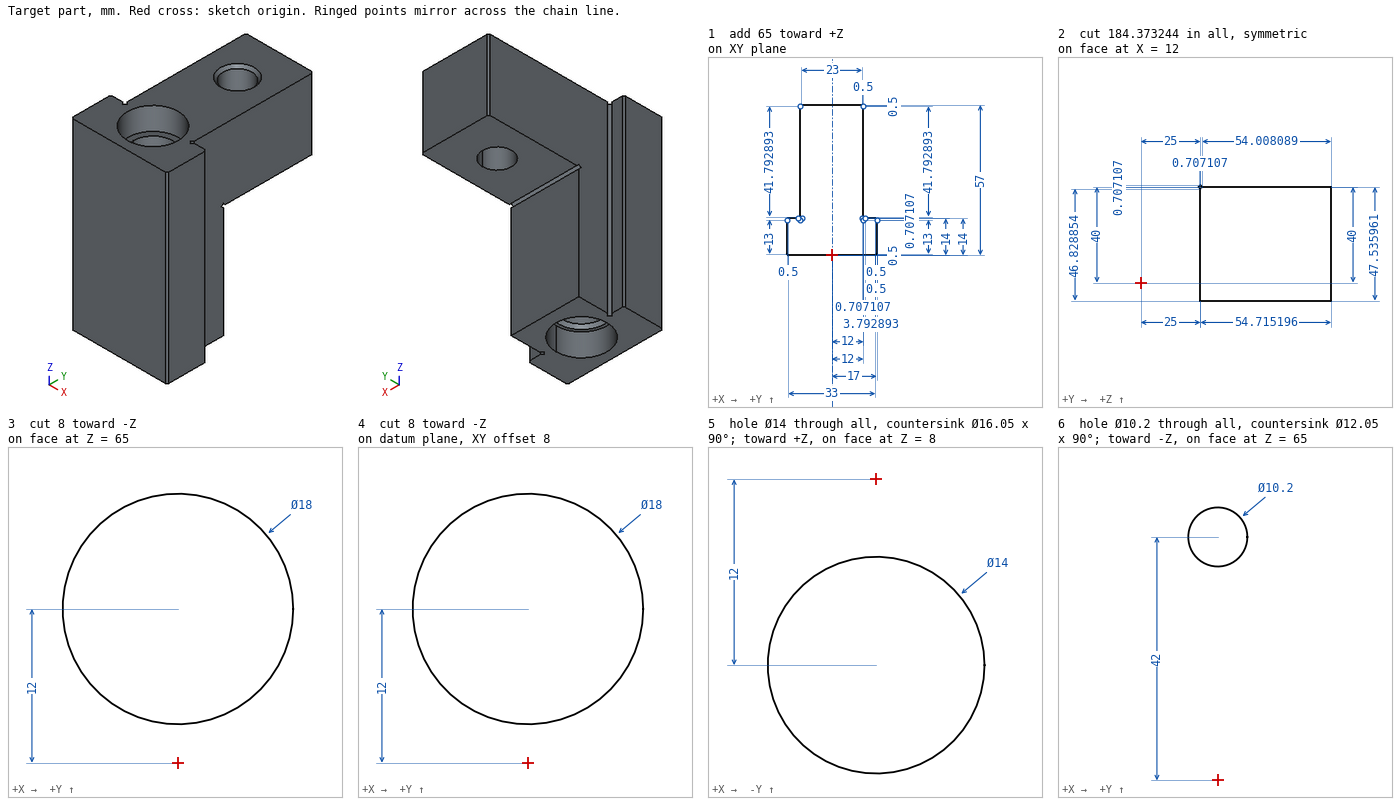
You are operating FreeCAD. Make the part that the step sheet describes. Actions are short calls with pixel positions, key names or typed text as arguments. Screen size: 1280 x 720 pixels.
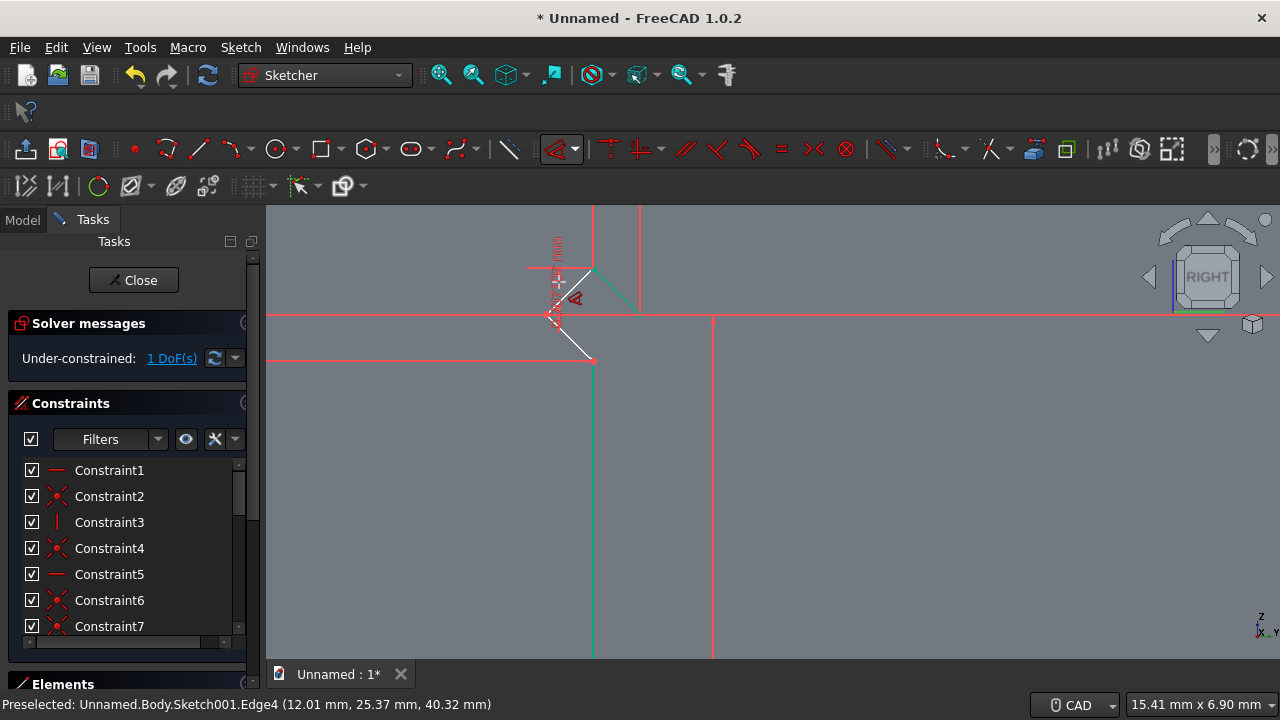
click(579, 282)
click(570, 234)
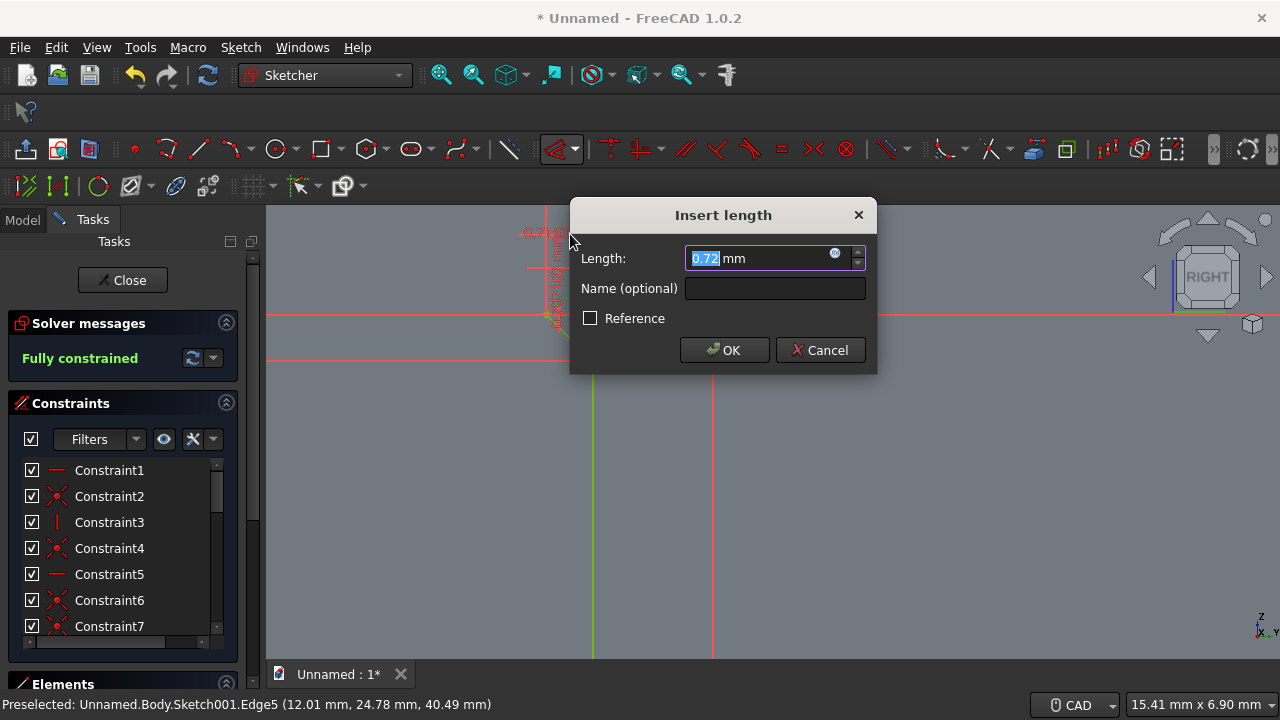
text(0.707107)
key(Return)
key(Escape)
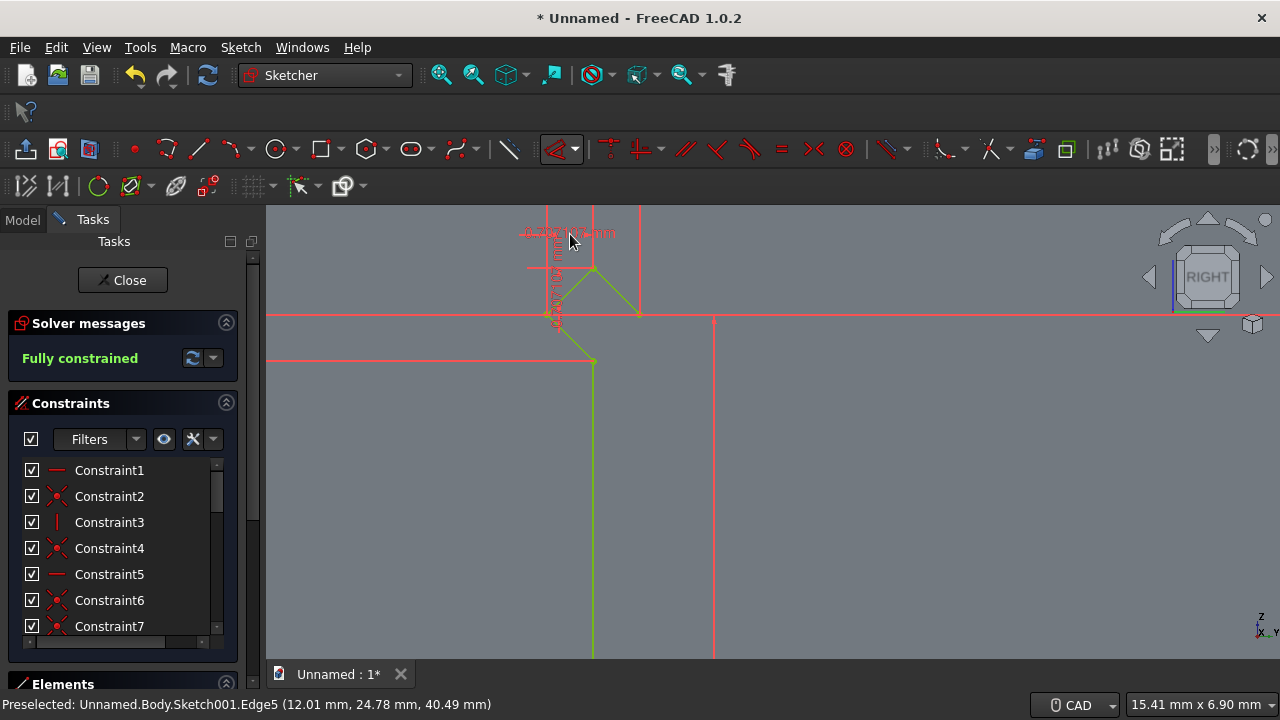
click(123, 280)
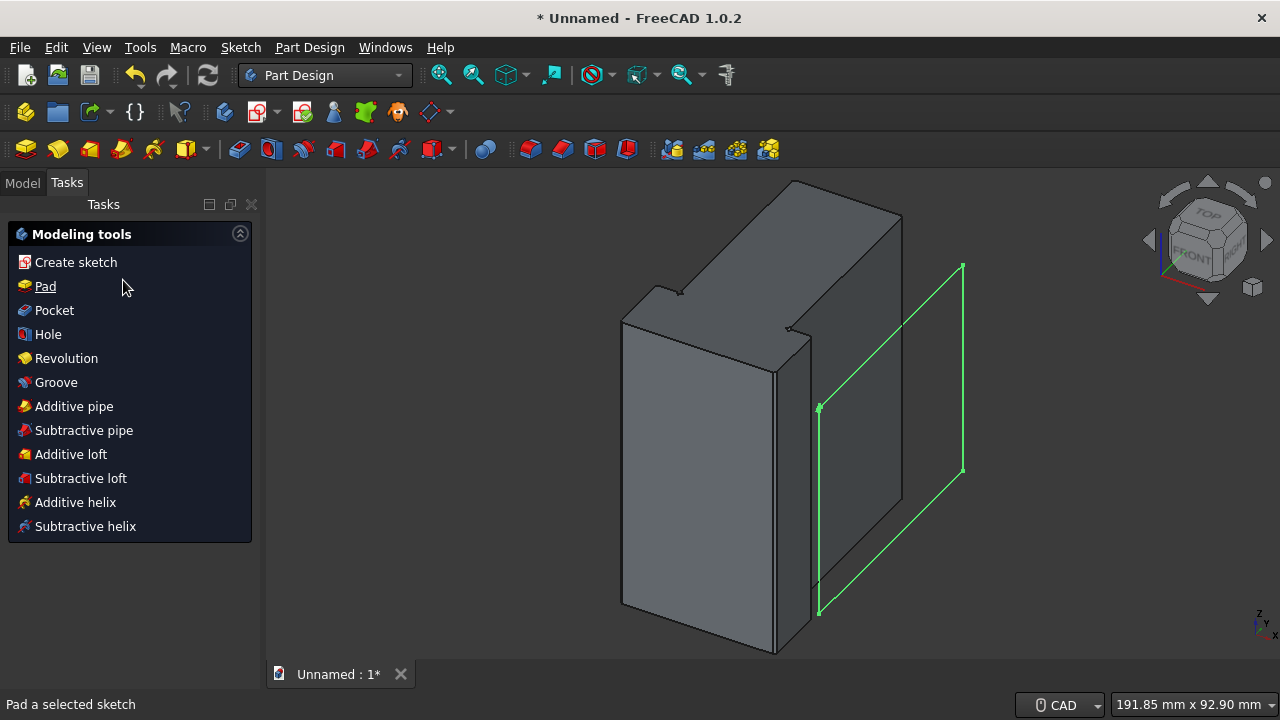
click(240, 150)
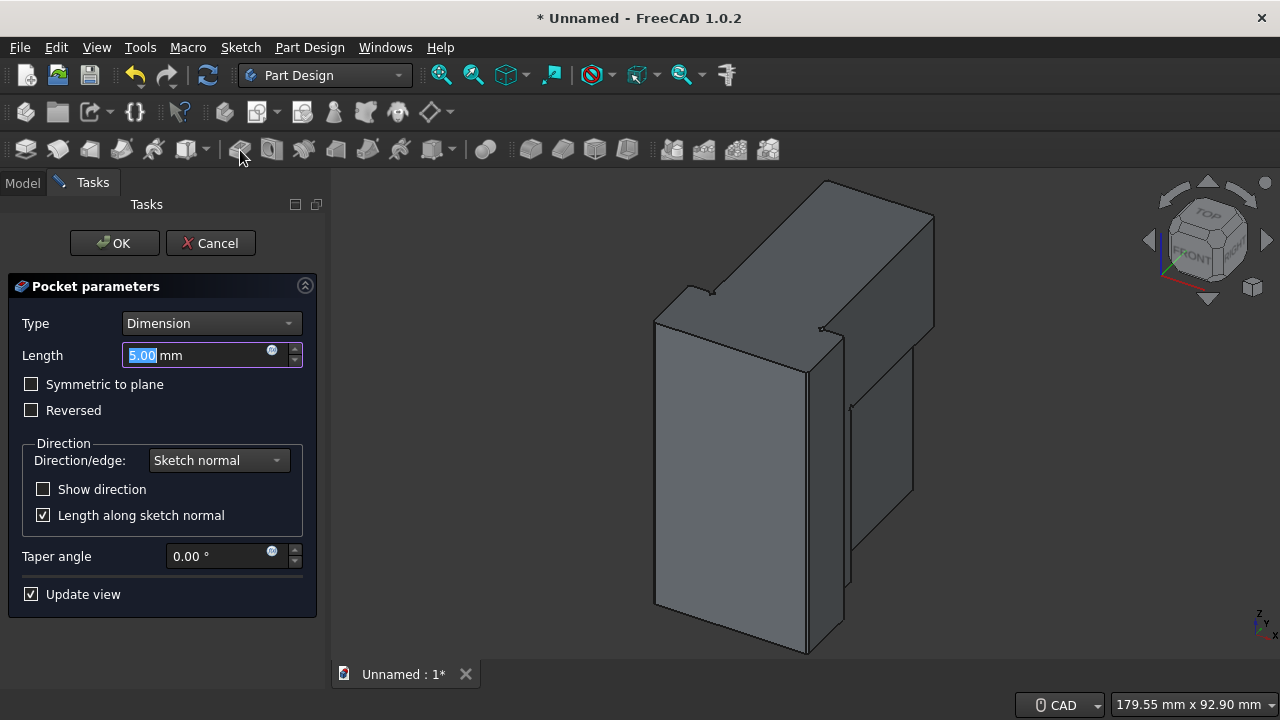
text(184.373244)
key(Tab)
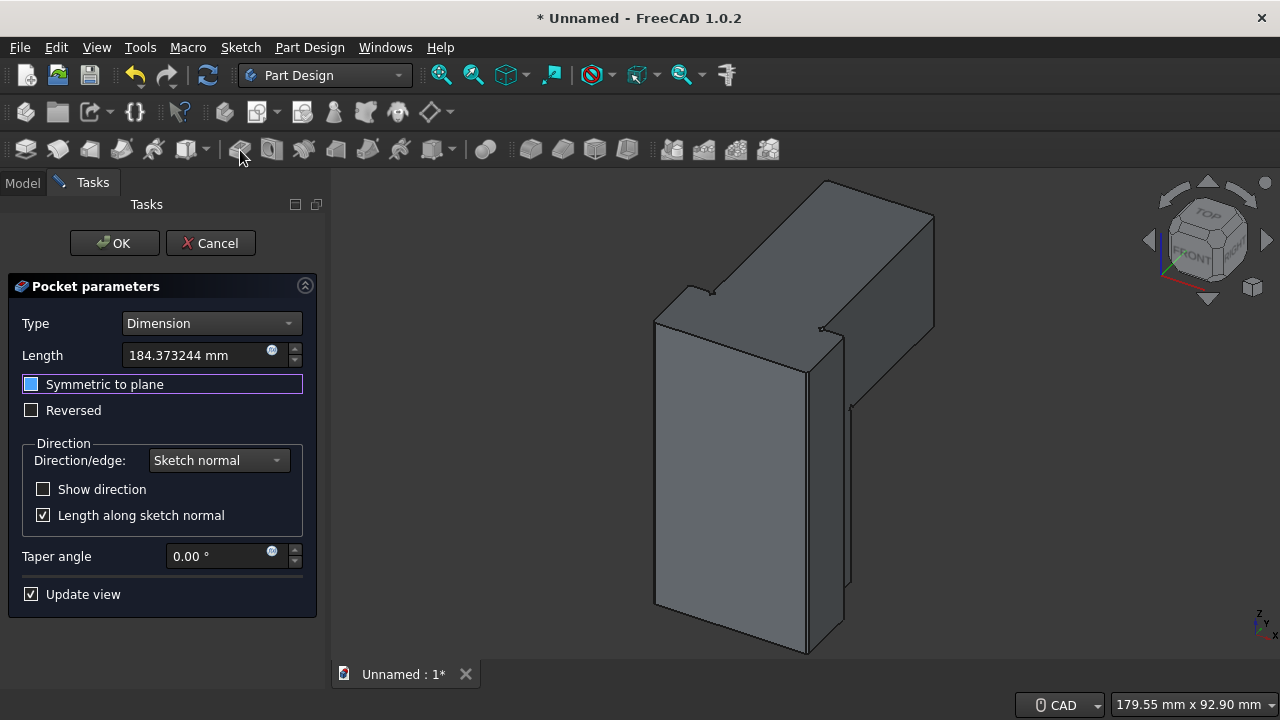
click(30, 384)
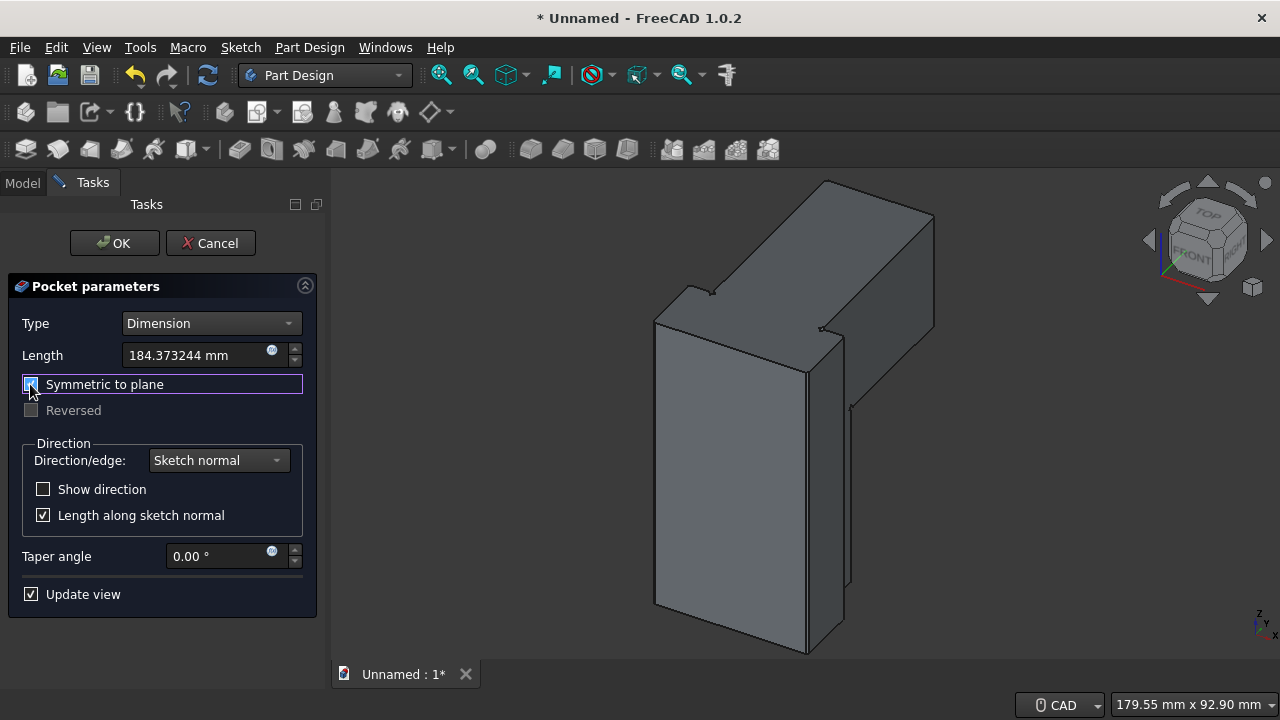
click(115, 243)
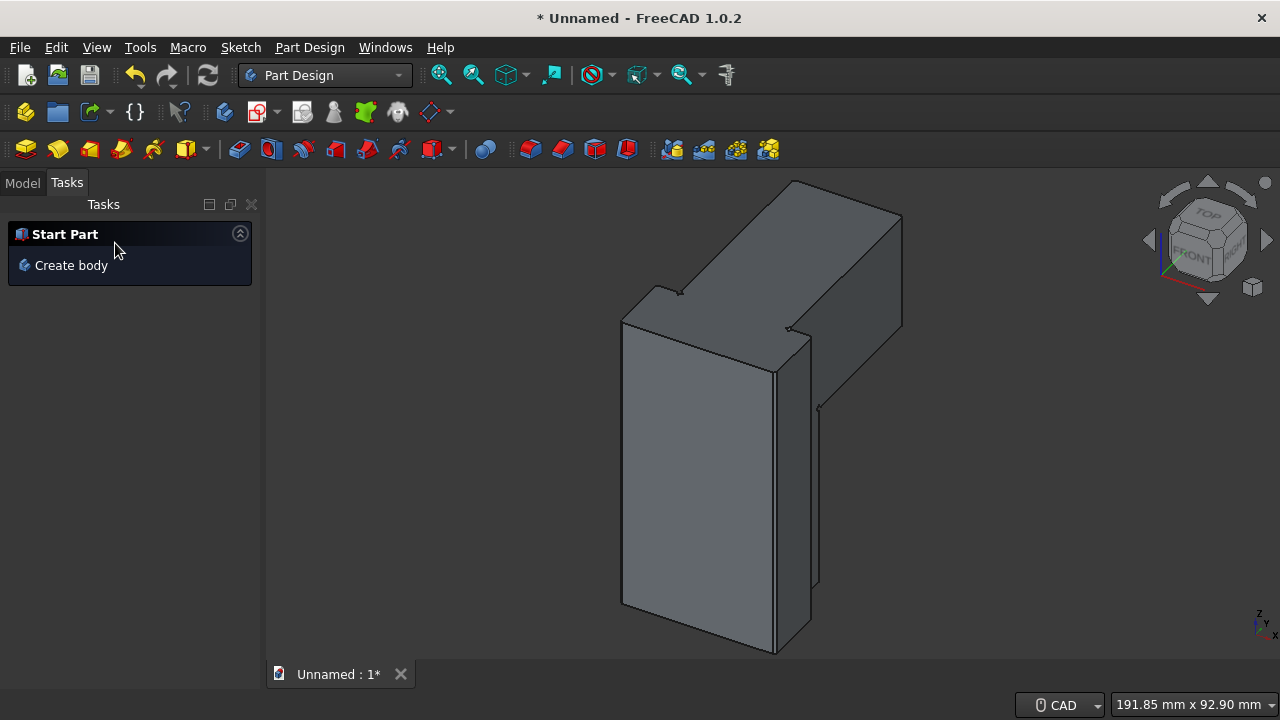
click(816, 229)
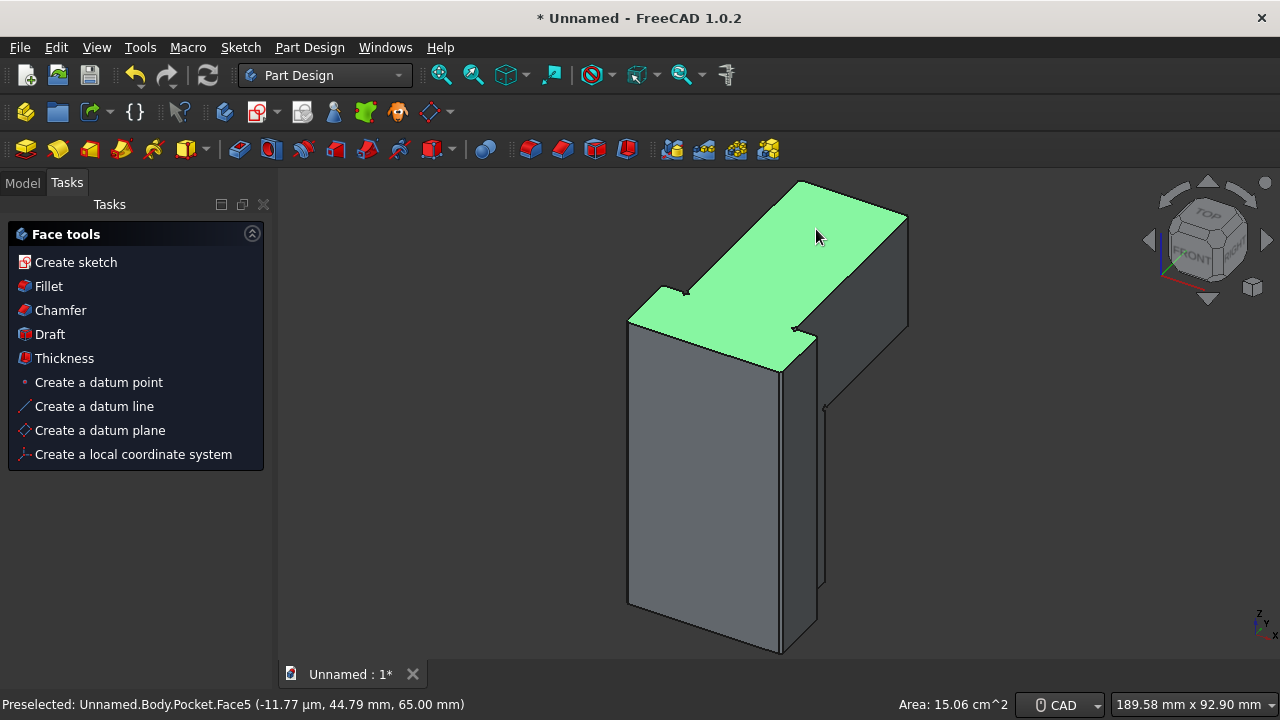
click(258, 112)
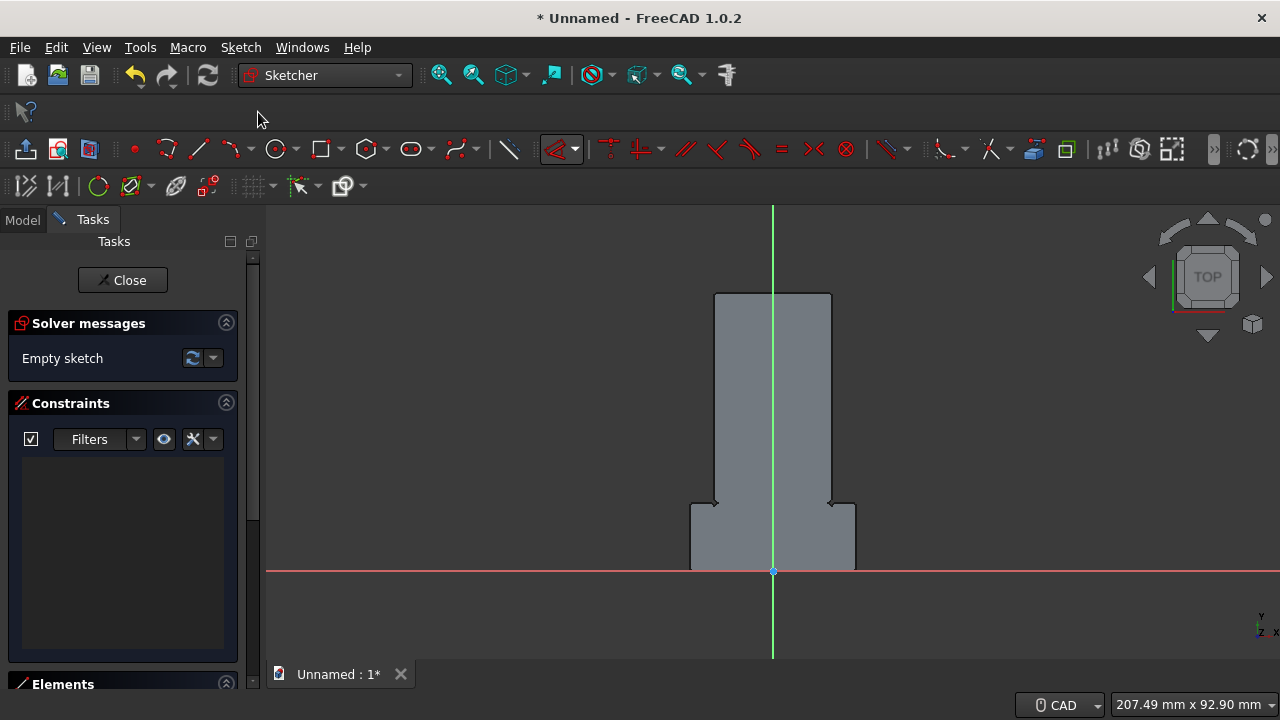
scroll(813, 571, up, 5)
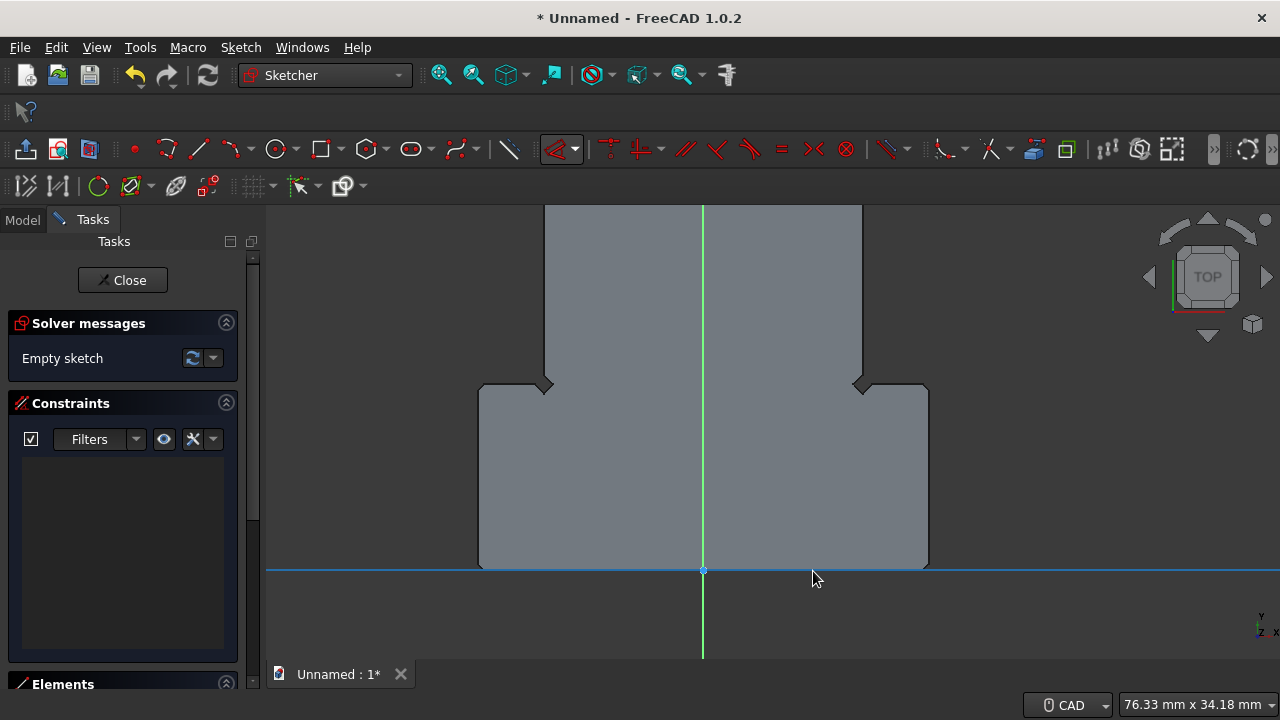
key(g)
key(c)